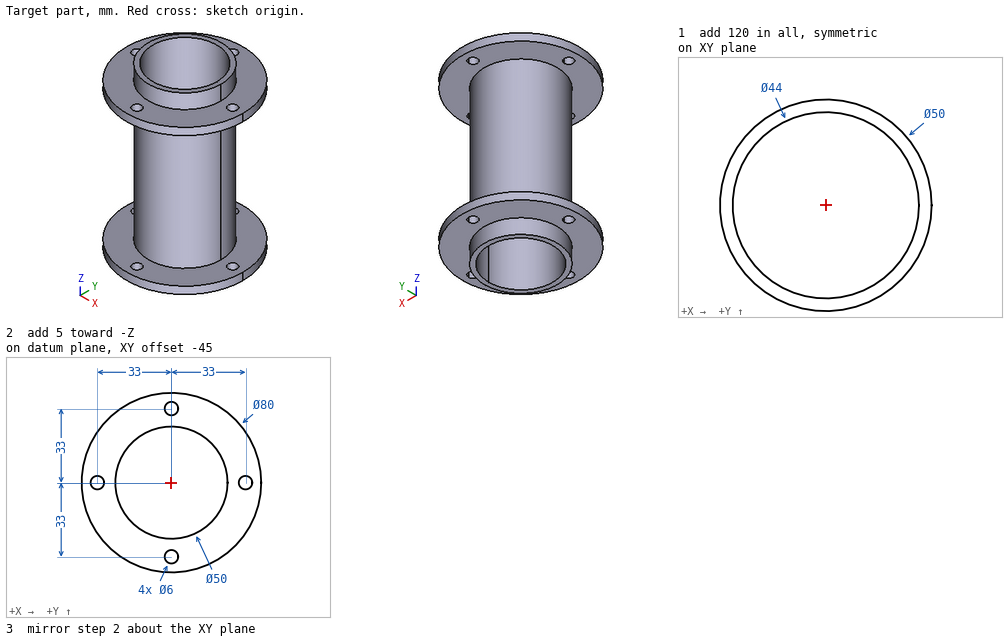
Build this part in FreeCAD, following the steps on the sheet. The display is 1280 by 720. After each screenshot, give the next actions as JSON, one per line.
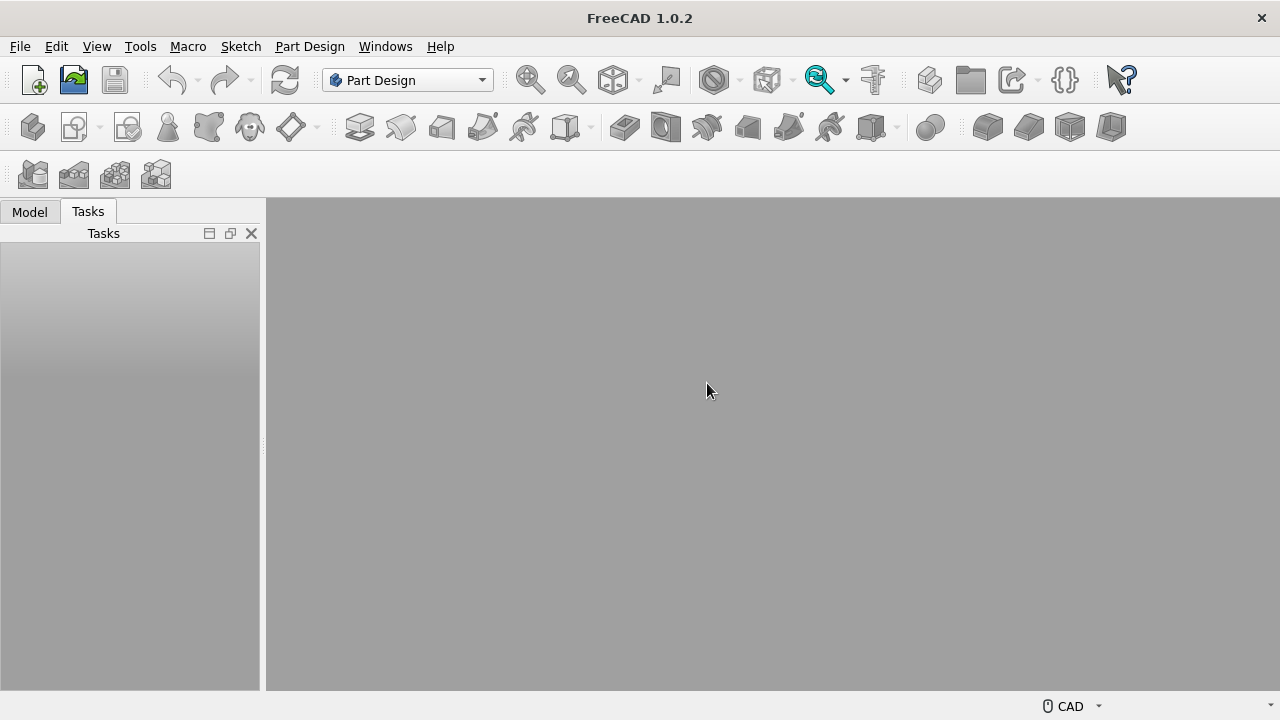
{"action": "left_click", "coordinate": [33, 80]}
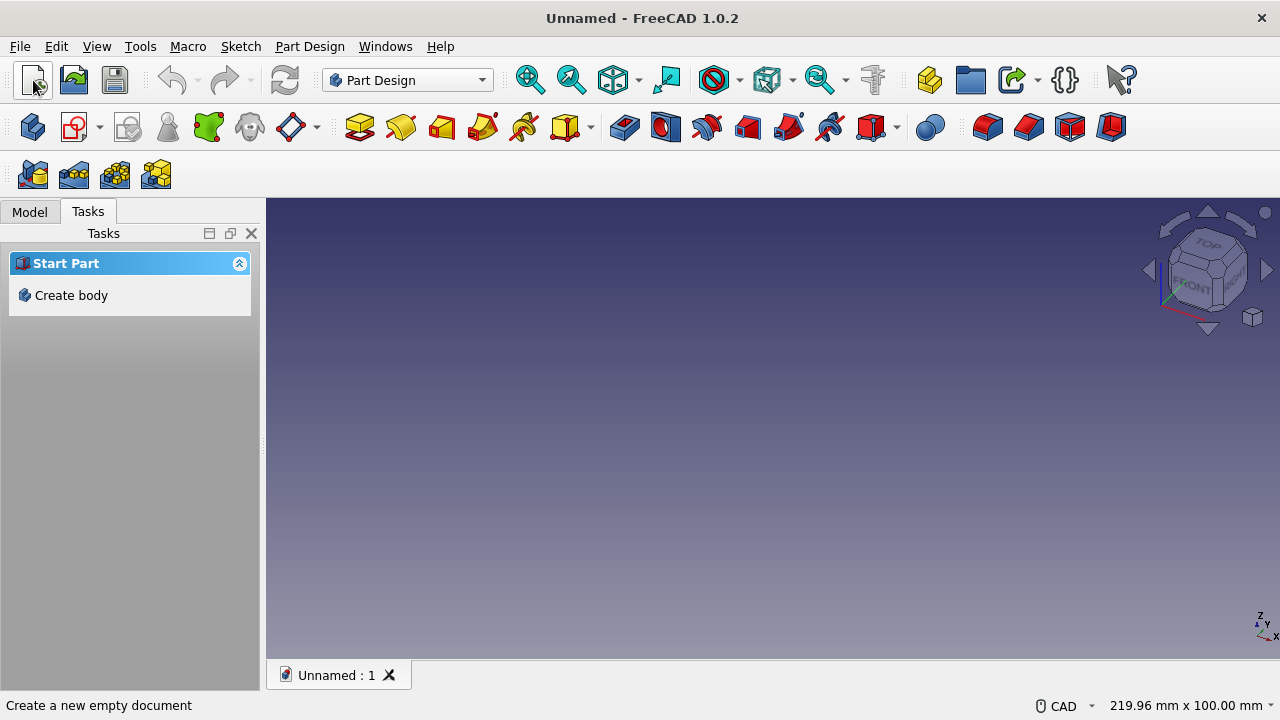
{"action": "left_click", "coordinate": [74, 128]}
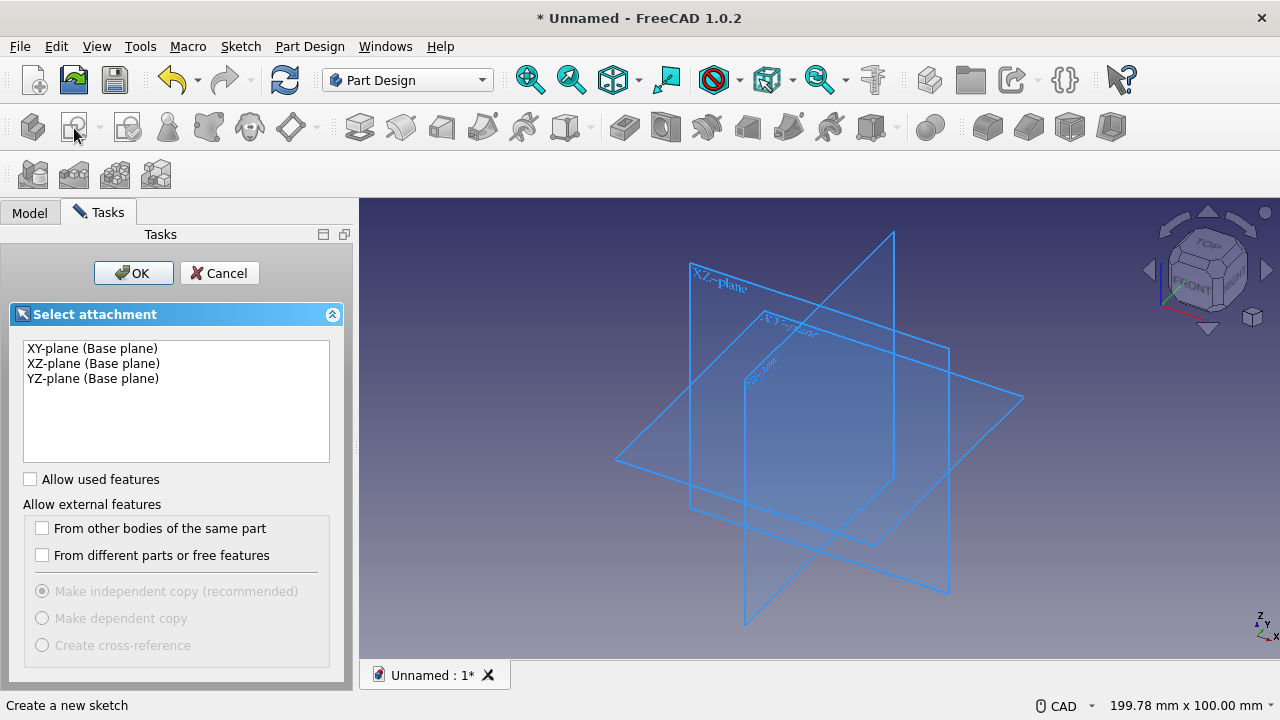
{"action": "left_click", "coordinate": [84, 348]}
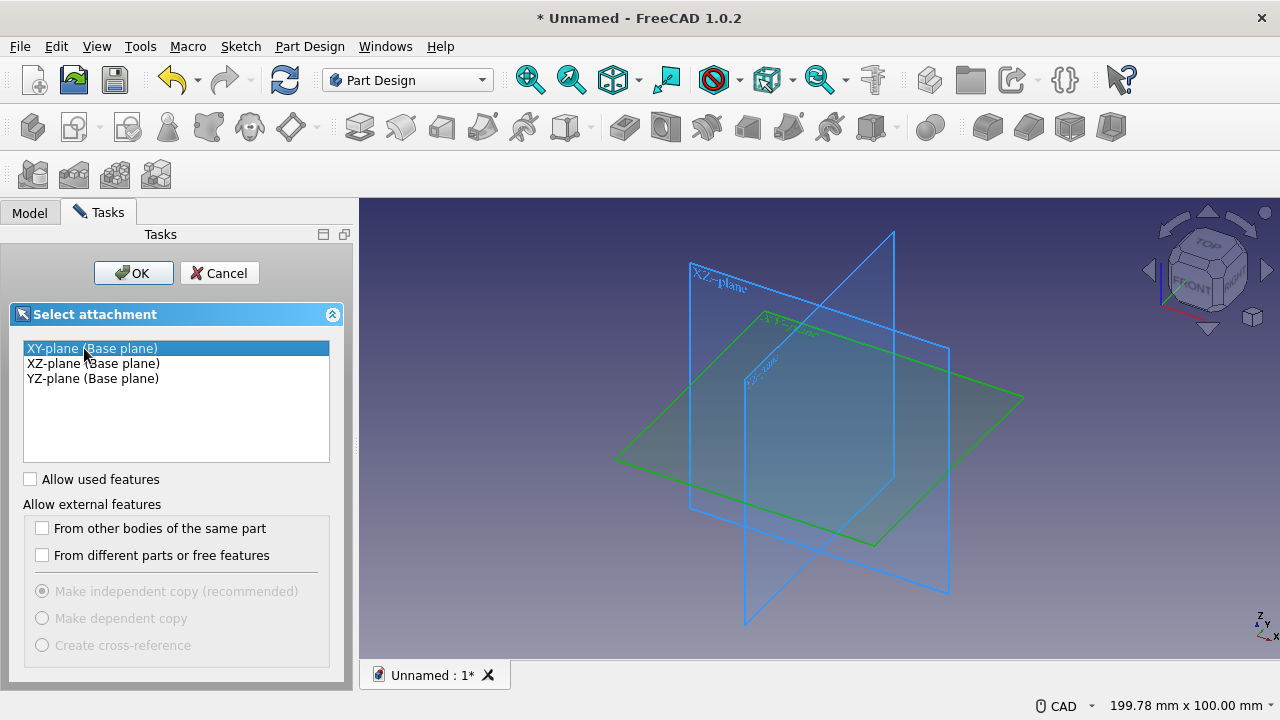
{"action": "left_click", "coordinate": [134, 273]}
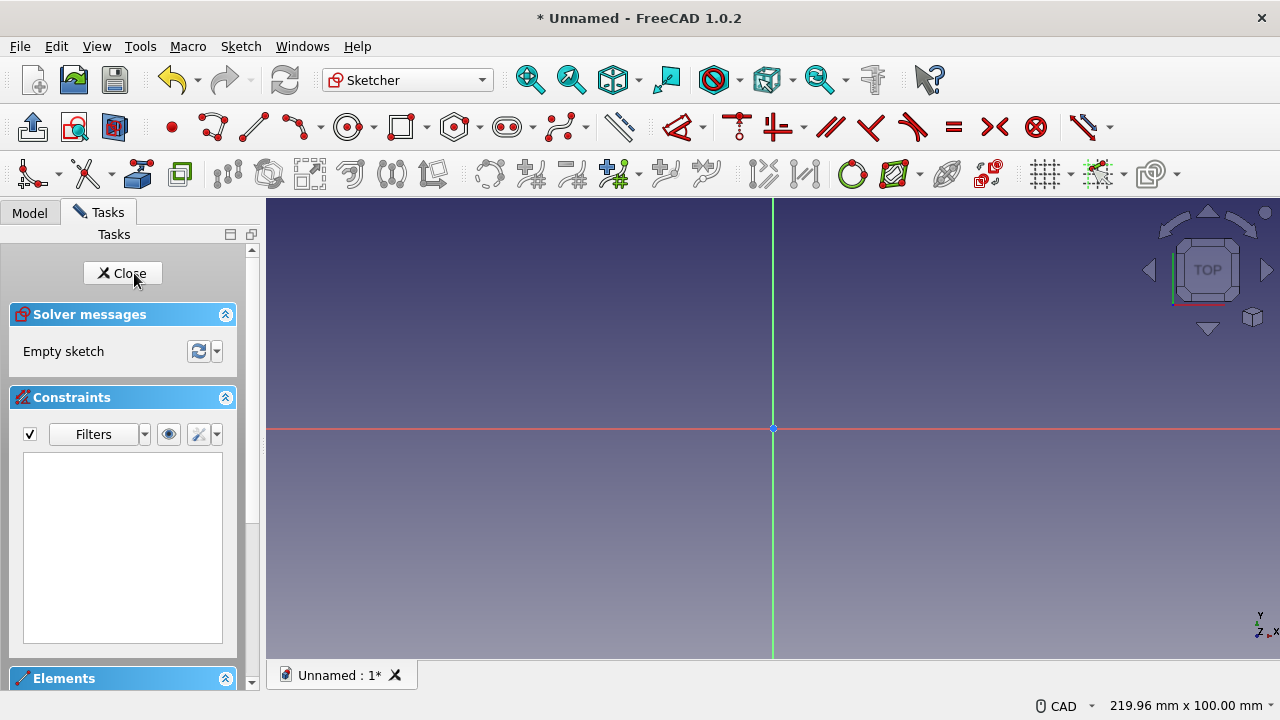
{"action": "left_click", "coordinate": [348, 128]}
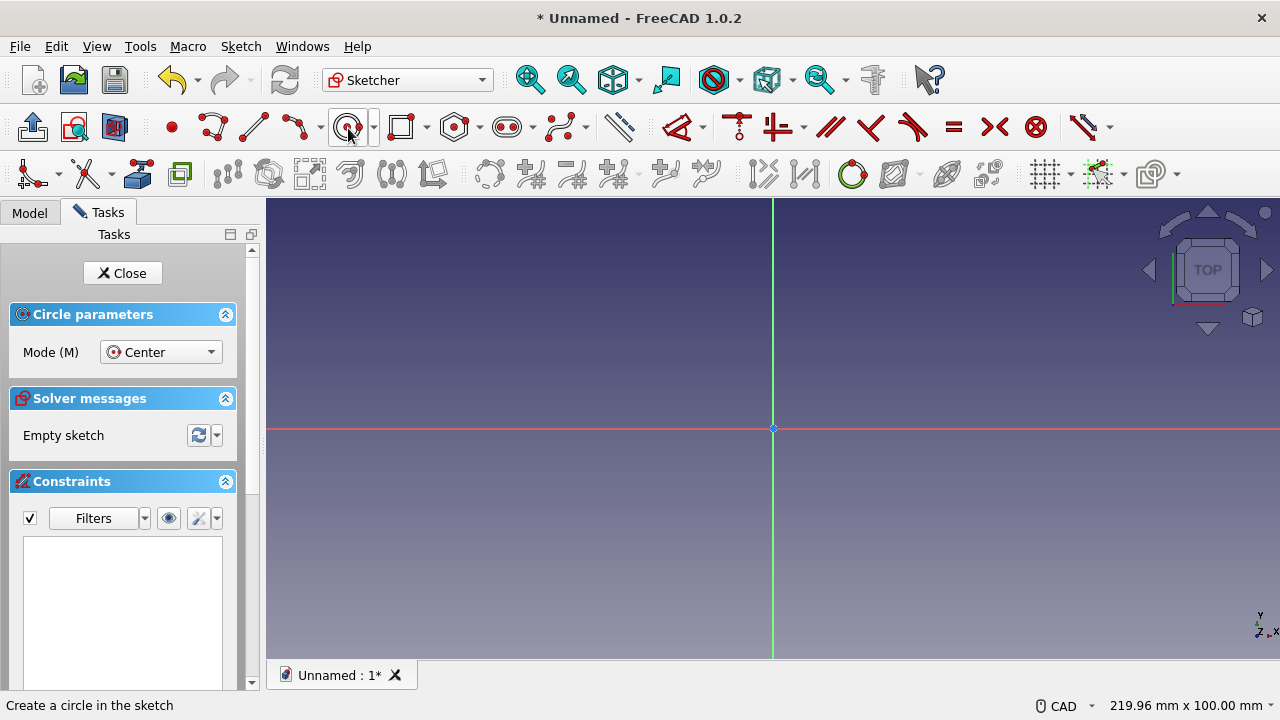
{"action": "left_click", "coordinate": [773, 428]}
{"action": "left_click", "coordinate": [854, 347]}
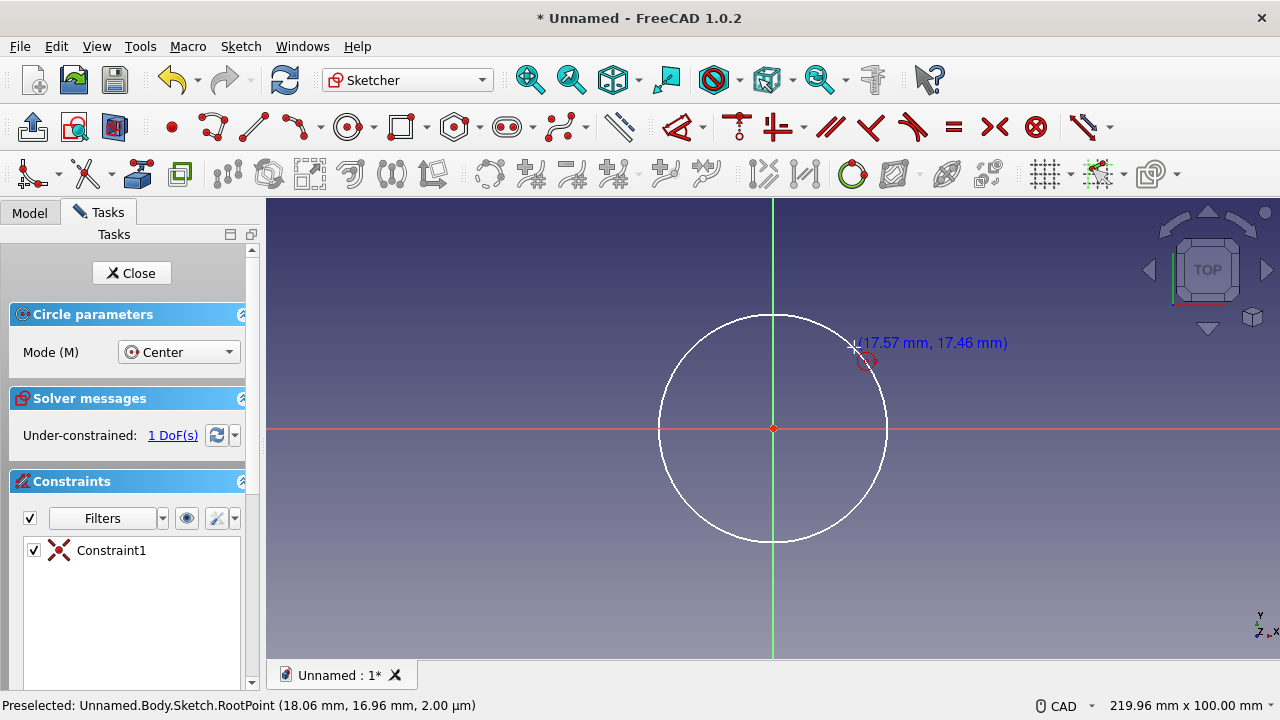
{"action": "left_click", "coordinate": [773, 428]}
{"action": "left_click", "coordinate": [845, 357]}
{"action": "key", "text": "Escape"}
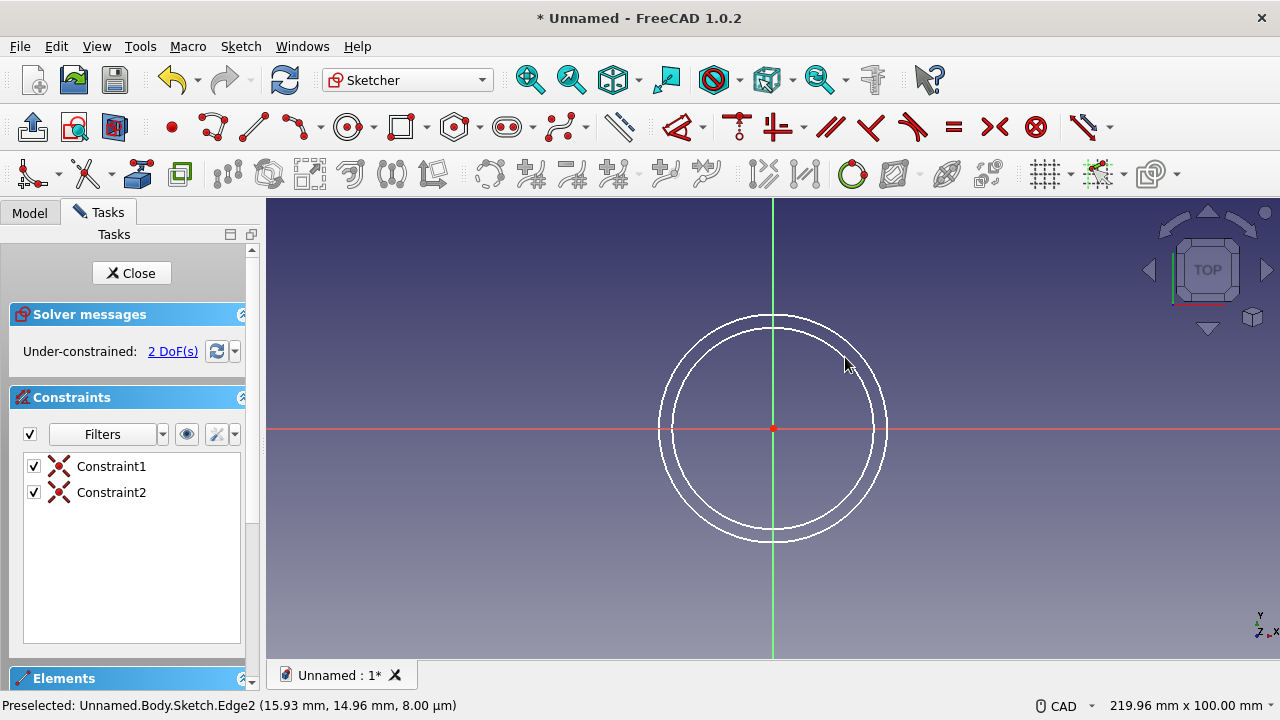
{"action": "left_click", "coordinate": [676, 128]}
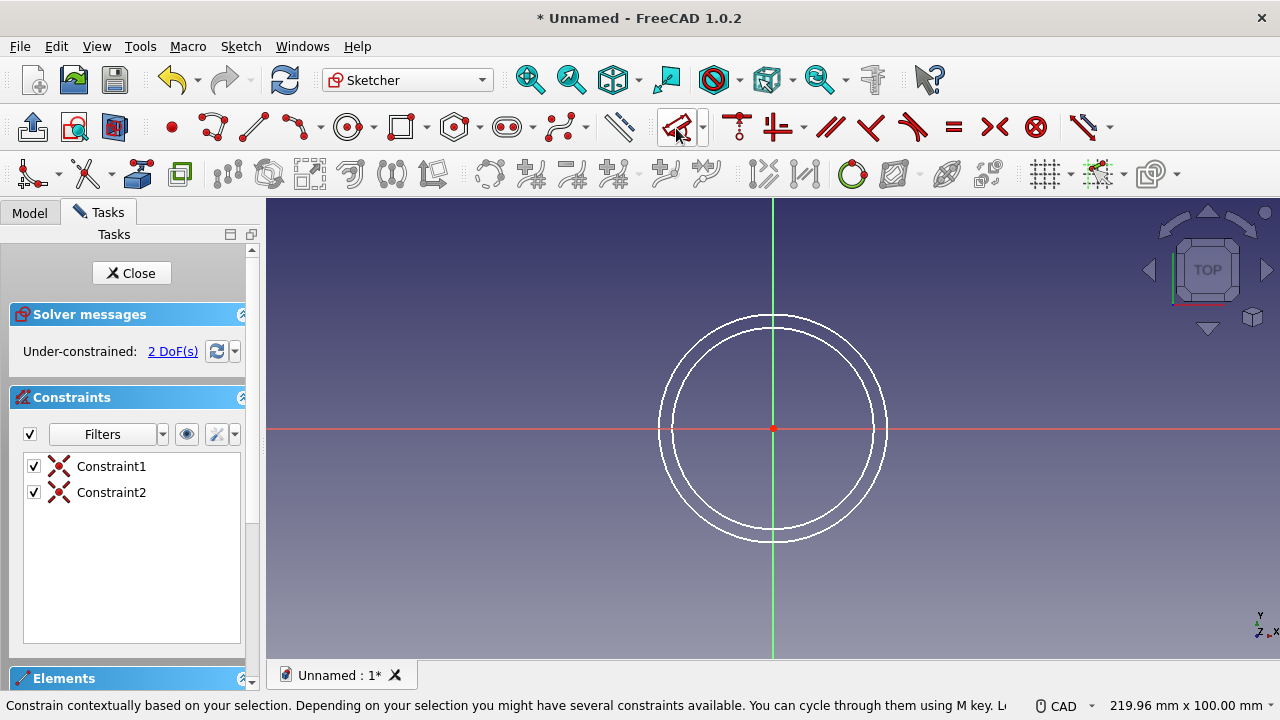
{"action": "left_click", "coordinate": [853, 347]}
{"action": "left_click", "coordinate": [875, 324]}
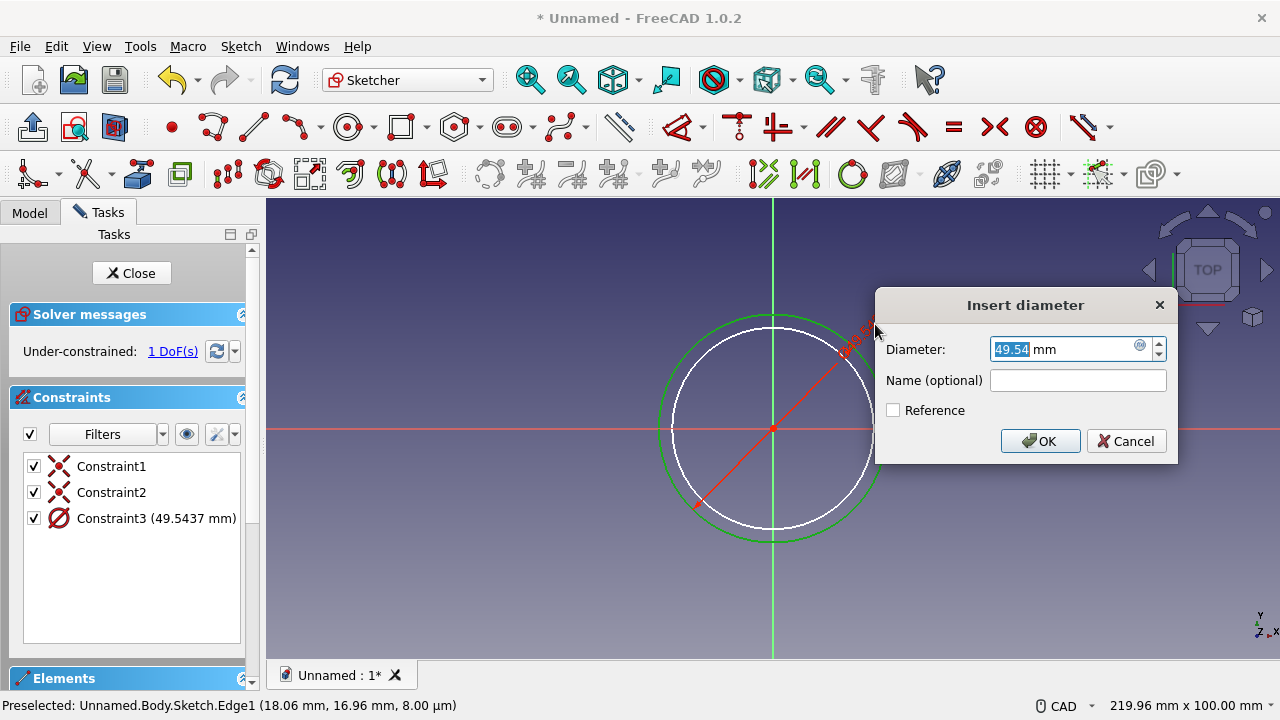
{"action": "type", "text": "50"}
{"action": "key", "text": "Return"}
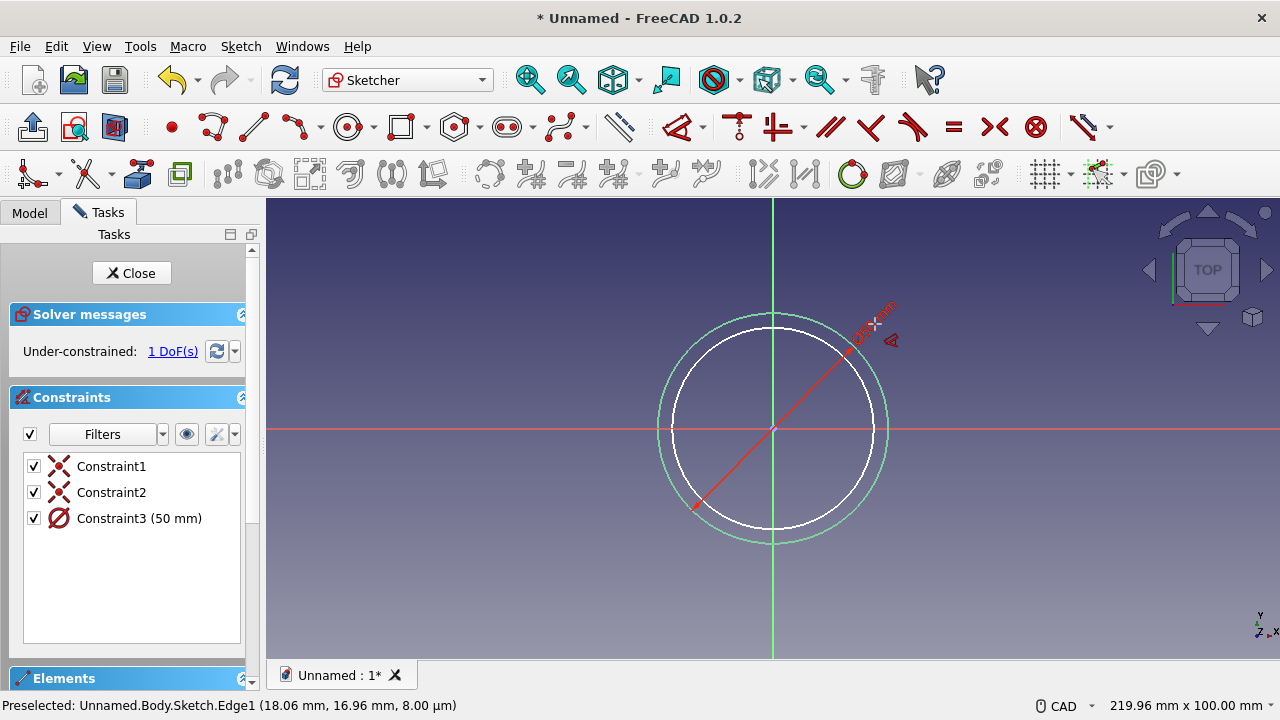
{"action": "left_click", "coordinate": [844, 357]}
{"action": "left_click", "coordinate": [900, 391]}